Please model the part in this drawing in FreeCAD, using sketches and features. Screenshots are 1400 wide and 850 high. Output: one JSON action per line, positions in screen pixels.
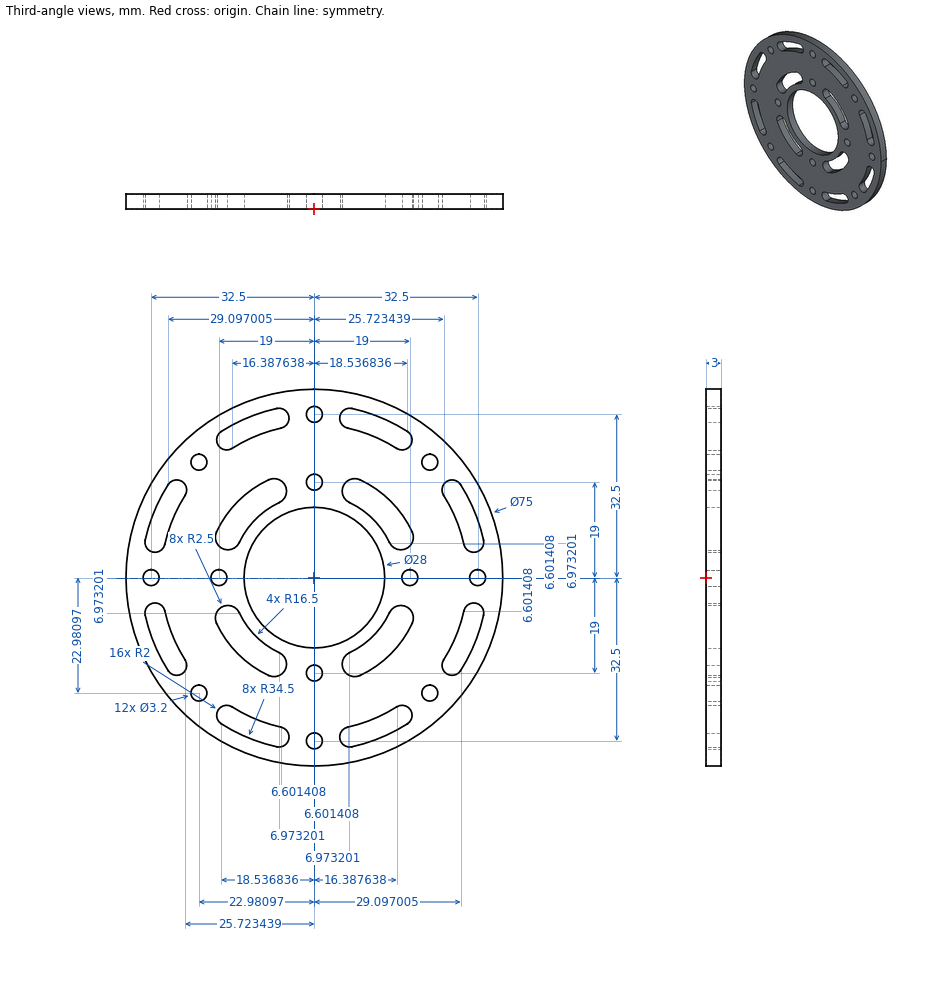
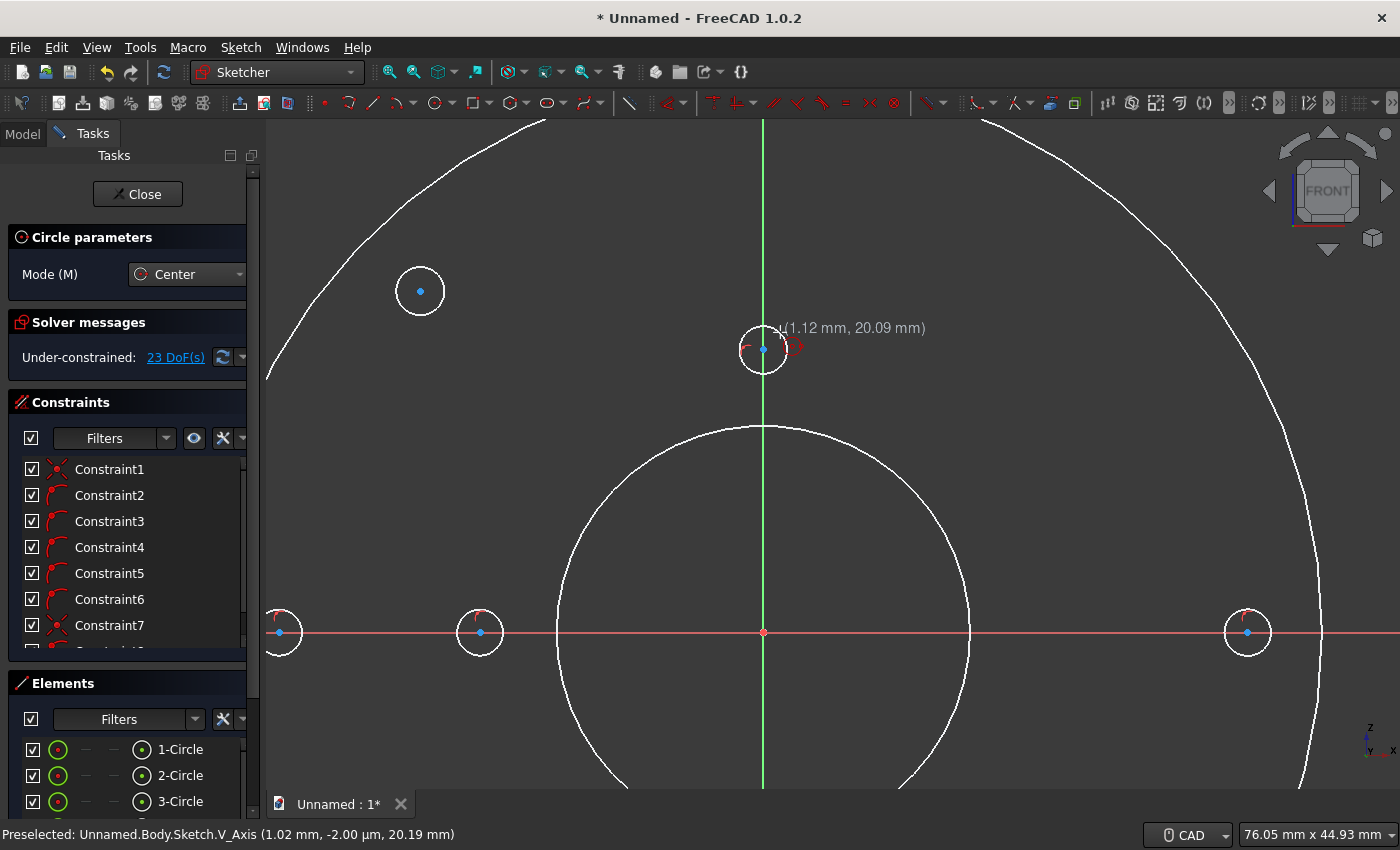
{"action": "left_click", "coordinate": [763, 148]}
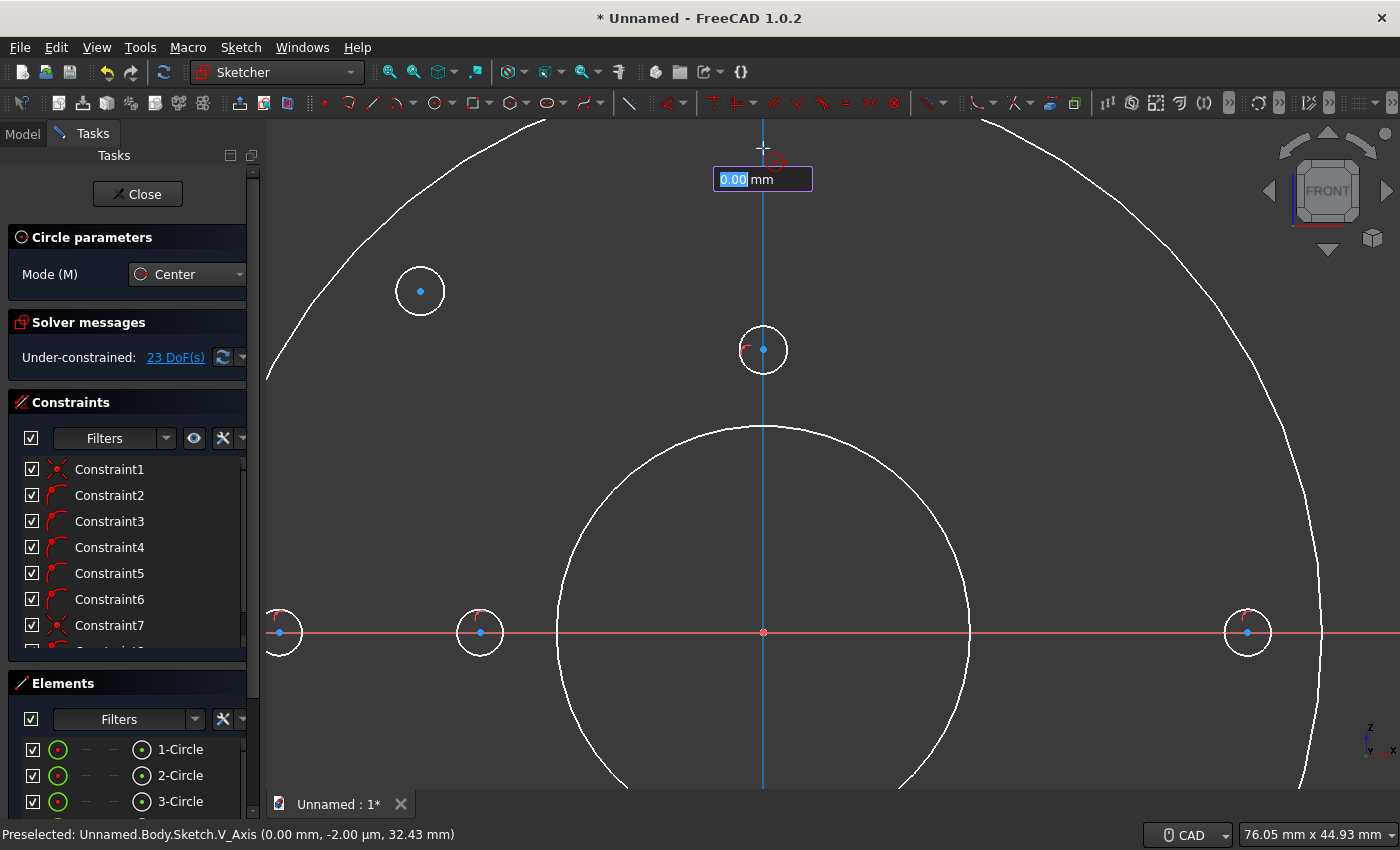
{"action": "scroll", "coordinate": [765, 350], "scroll_direction": "down", "scroll_amount": 5}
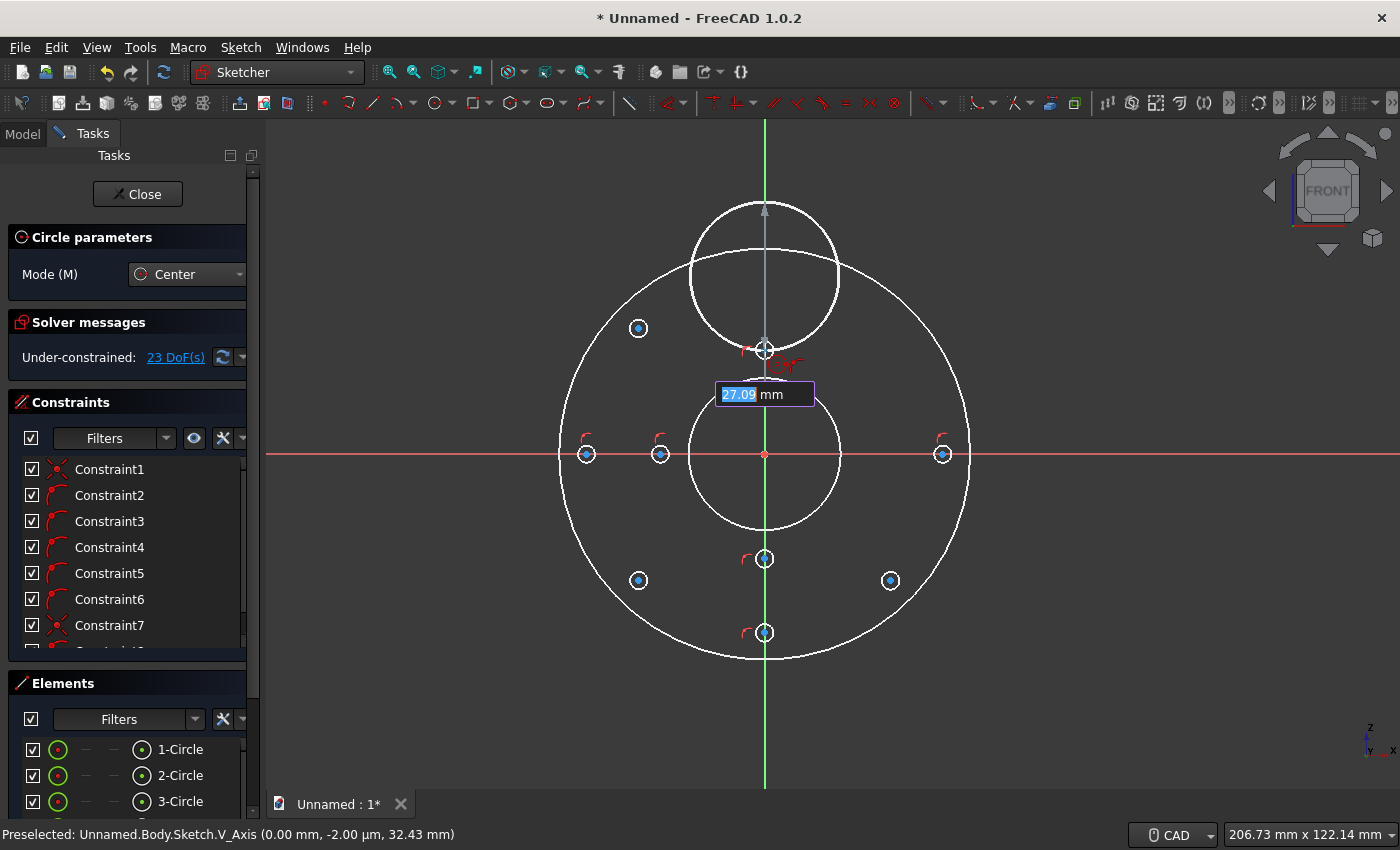
{"action": "scroll", "coordinate": [771, 270], "scroll_direction": "up", "scroll_amount": 5}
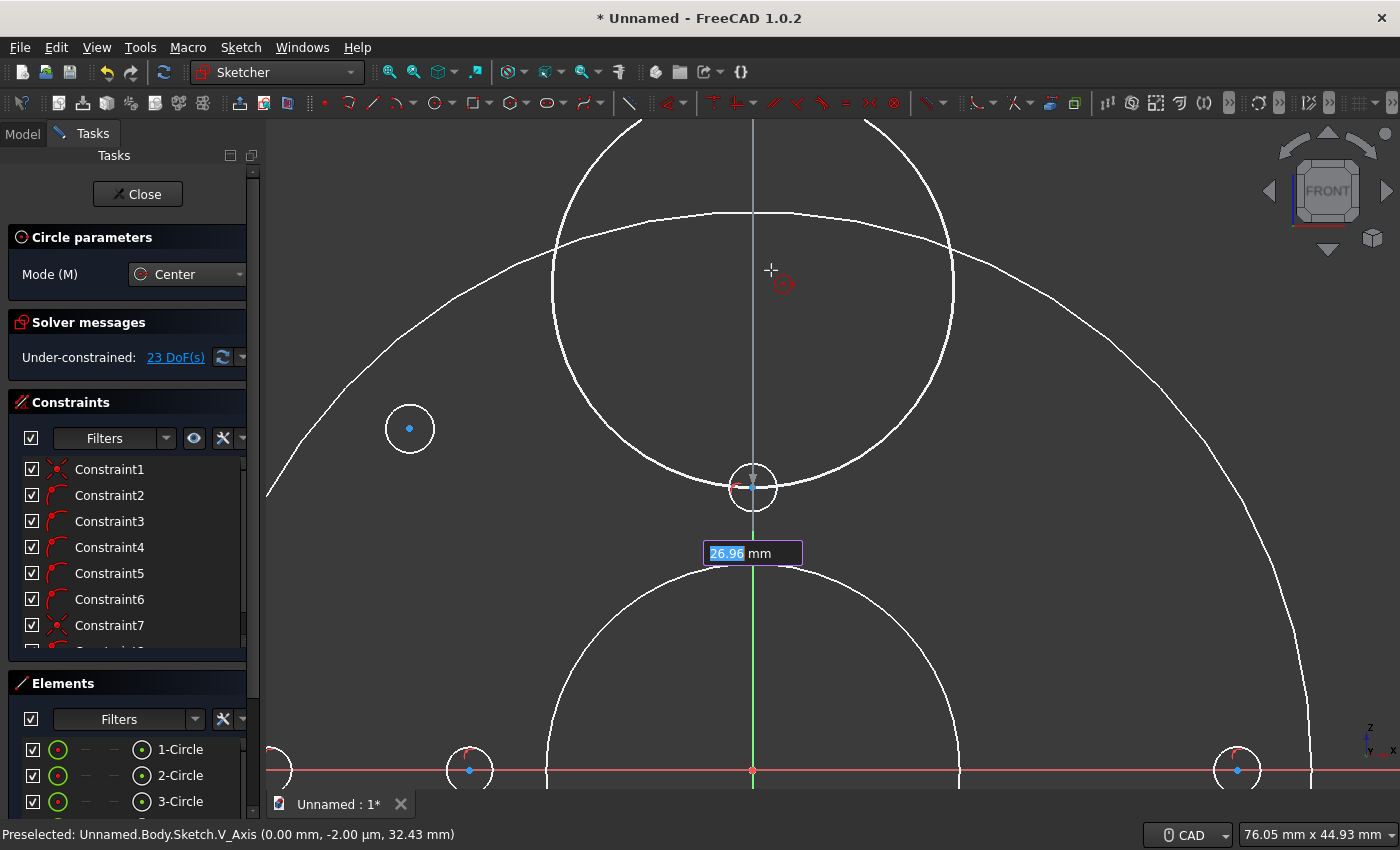
{"action": "left_click", "coordinate": [770, 269]}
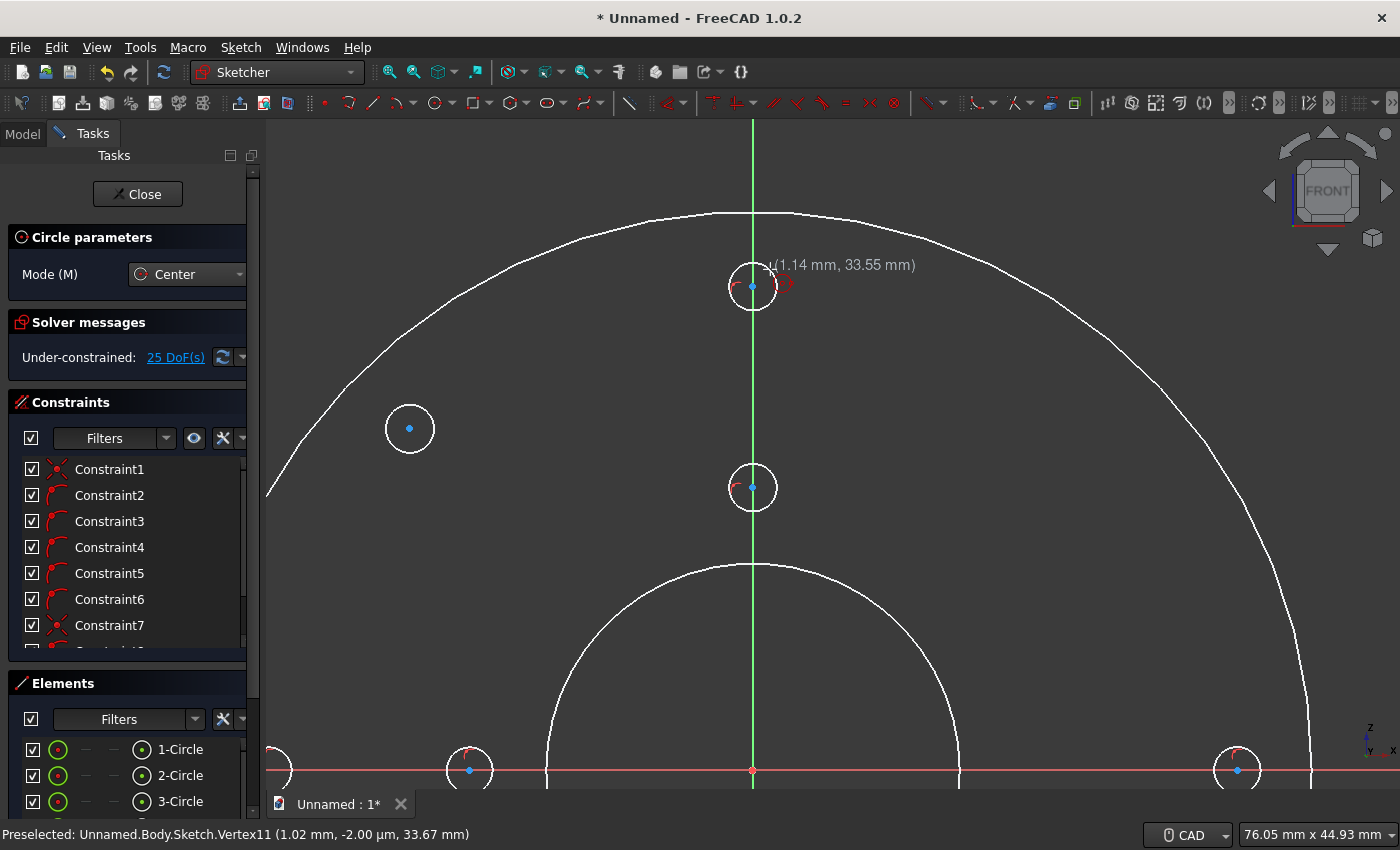
{"action": "scroll", "coordinate": [771, 270], "scroll_direction": "down", "scroll_amount": 5}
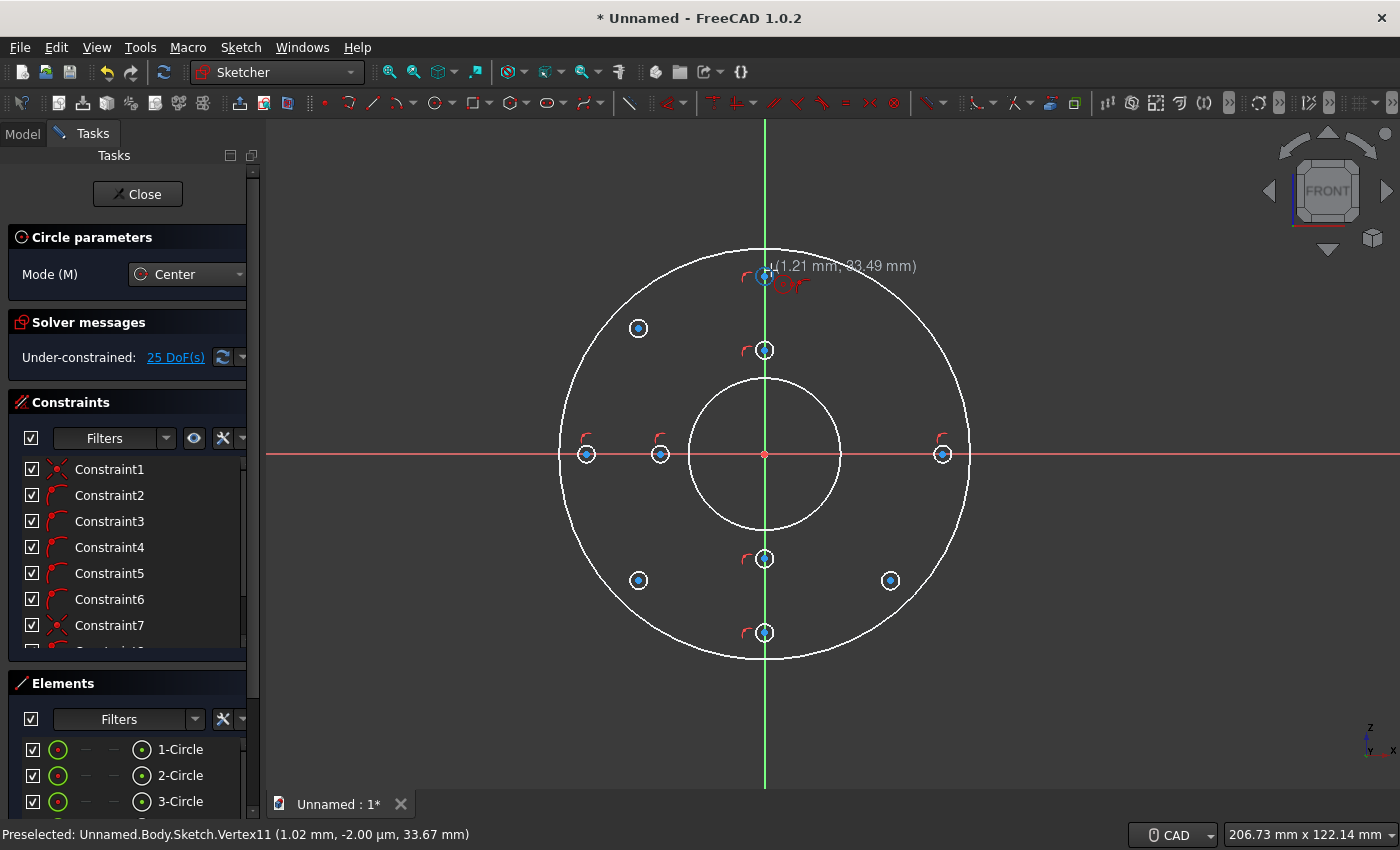
{"action": "scroll", "coordinate": [869, 454], "scroll_direction": "up", "scroll_amount": 5}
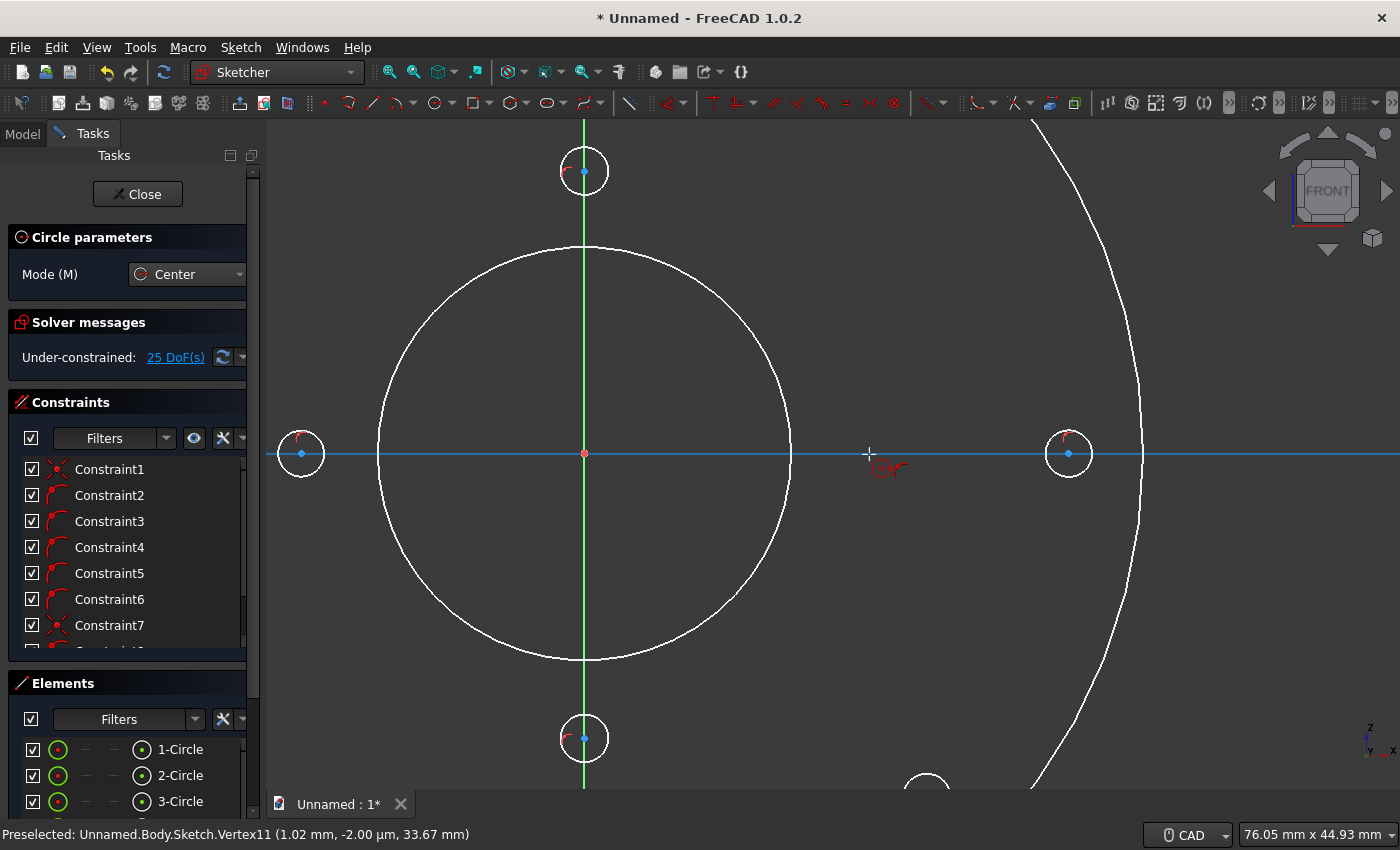
{"action": "left_click", "coordinate": [868, 454]}
{"action": "left_click", "coordinate": [885, 437]}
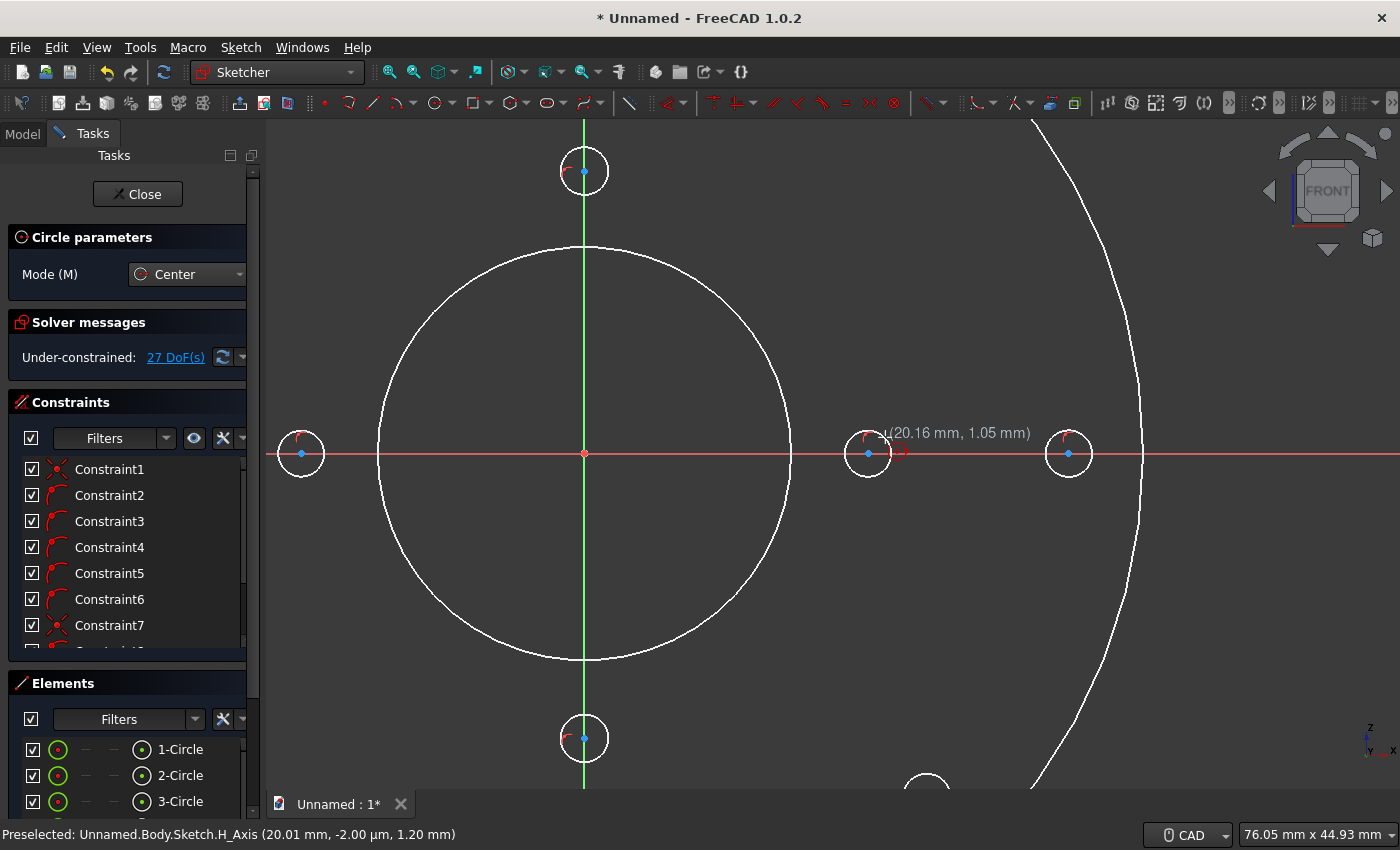
{"action": "scroll", "coordinate": [869, 454], "scroll_direction": "down", "scroll_amount": 5}